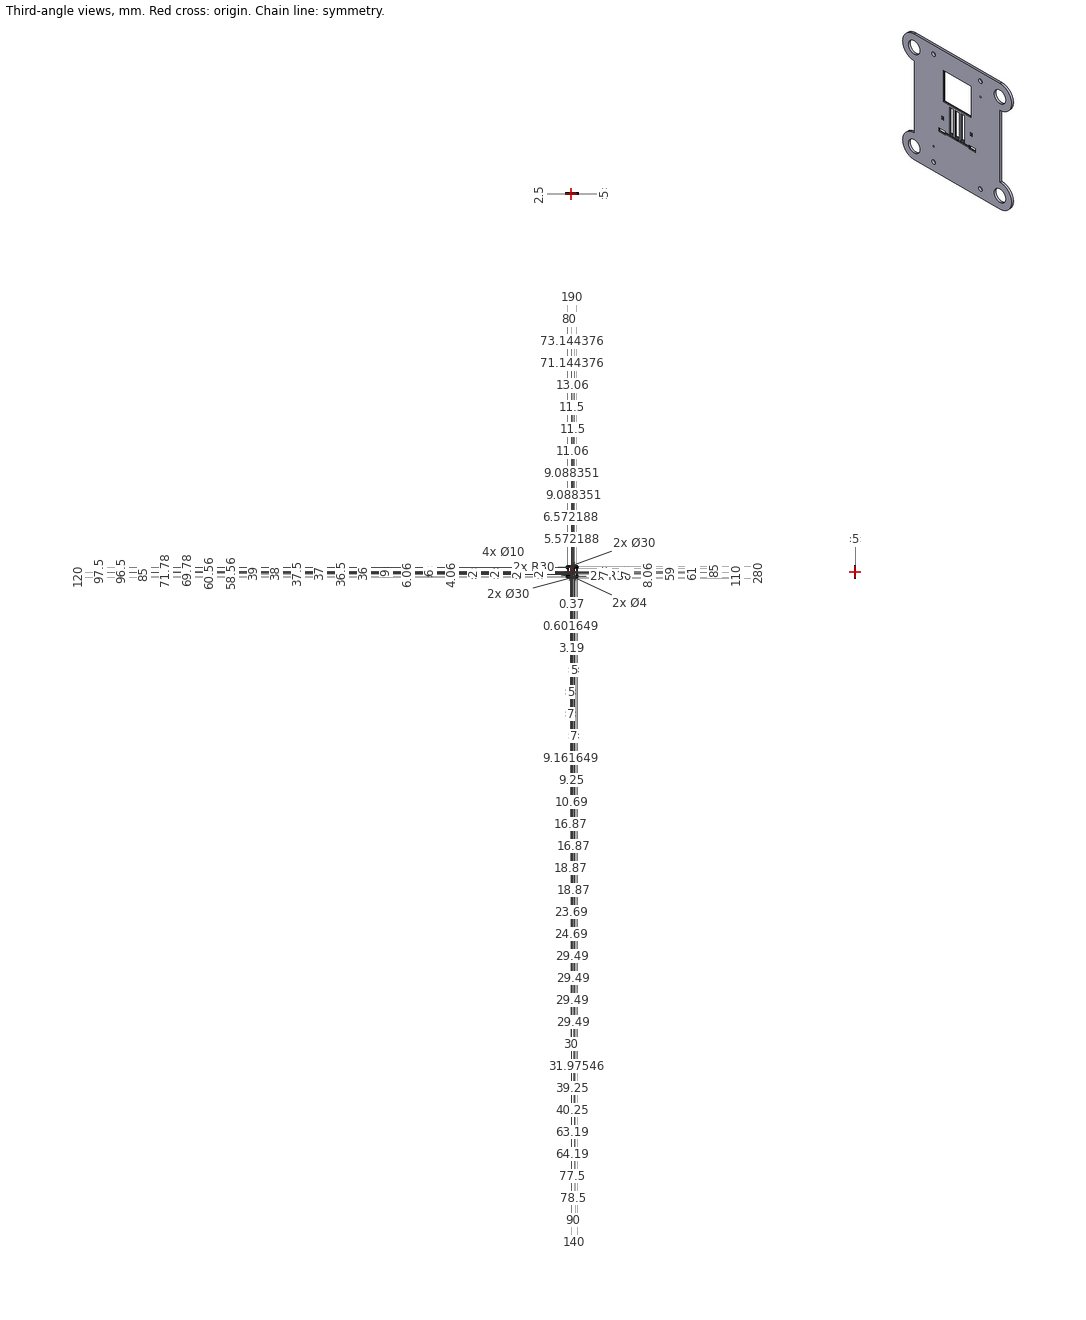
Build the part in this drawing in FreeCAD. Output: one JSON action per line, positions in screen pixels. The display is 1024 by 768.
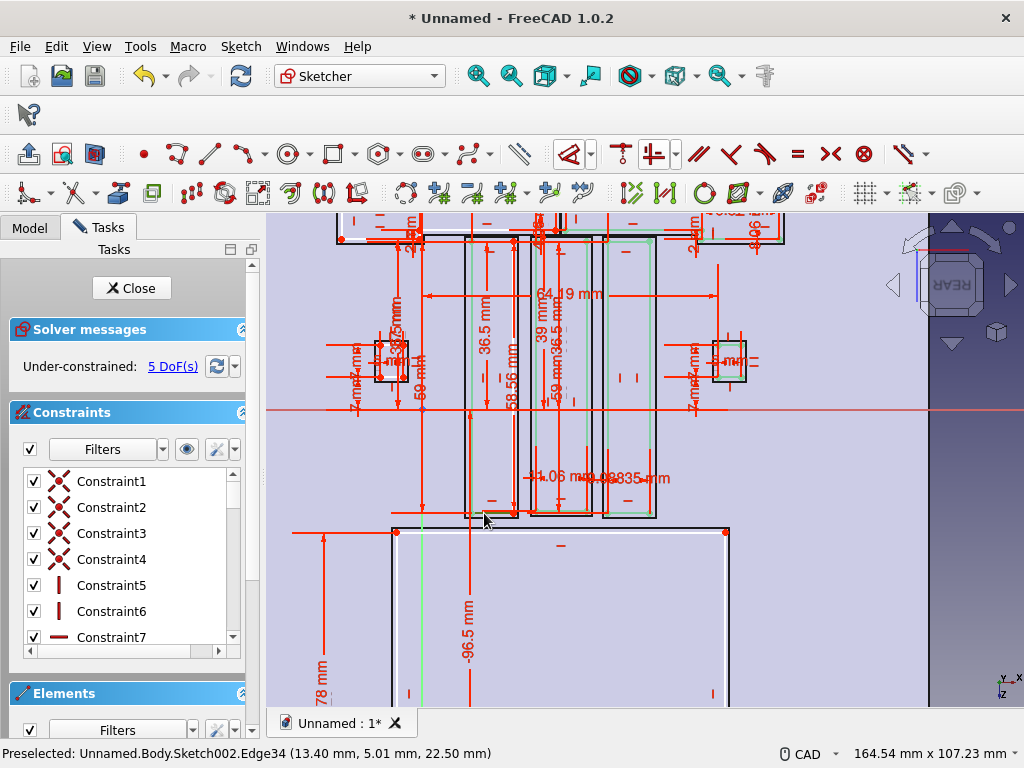
{"action": "key", "text": "l"}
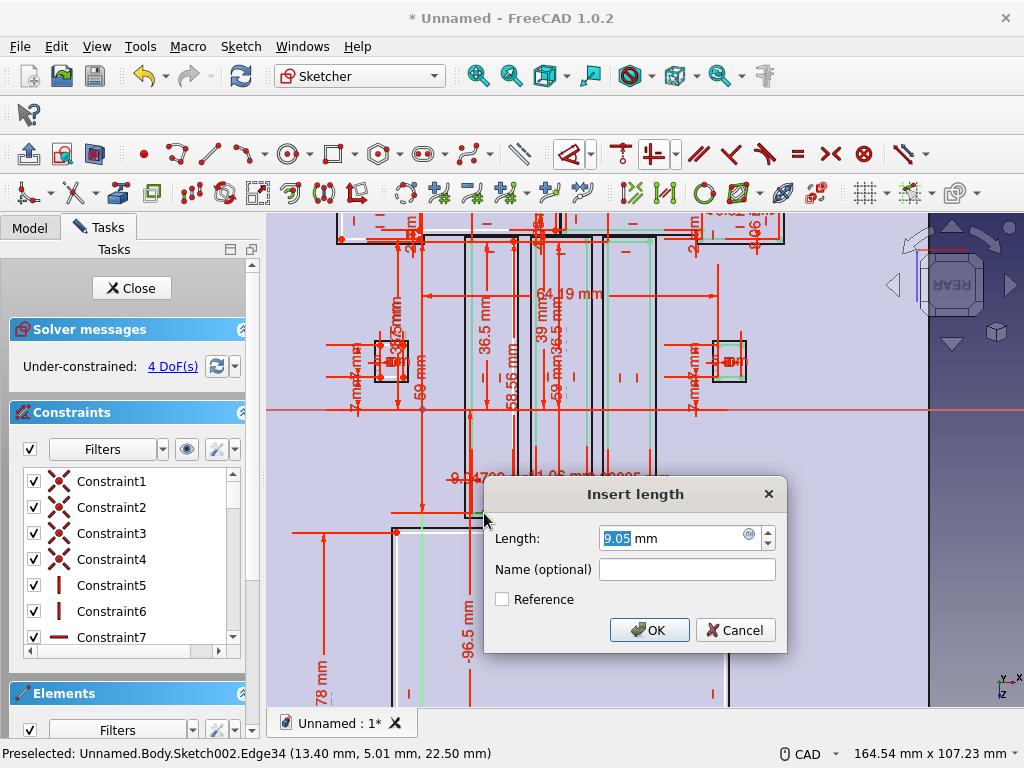
{"action": "type", "text": "9.088351"}
{"action": "key", "text": "Return"}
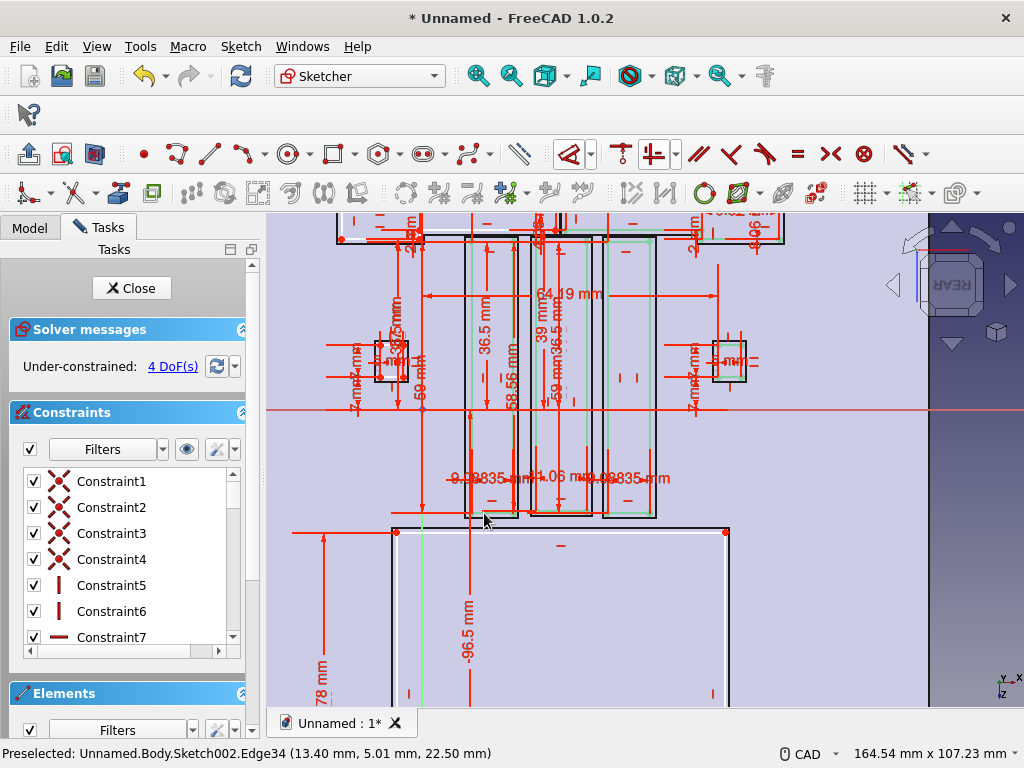
{"action": "scroll", "coordinate": [590, 404], "scroll_direction": "down", "scroll_amount": 4}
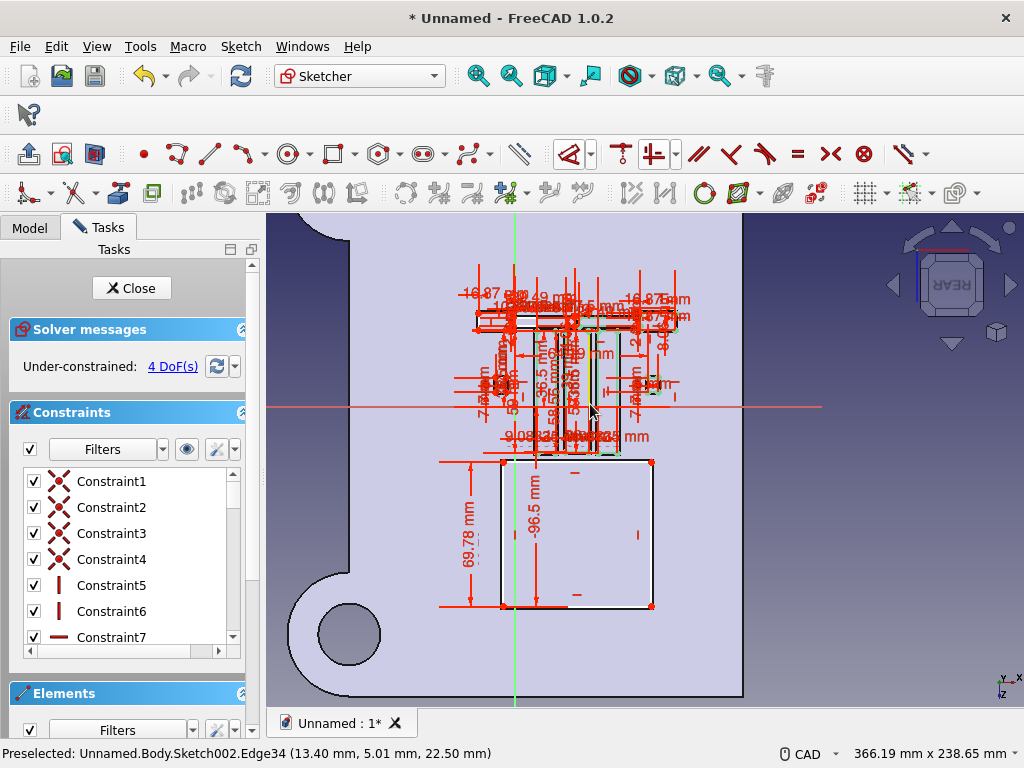
{"action": "left_click", "coordinate": [548, 607]}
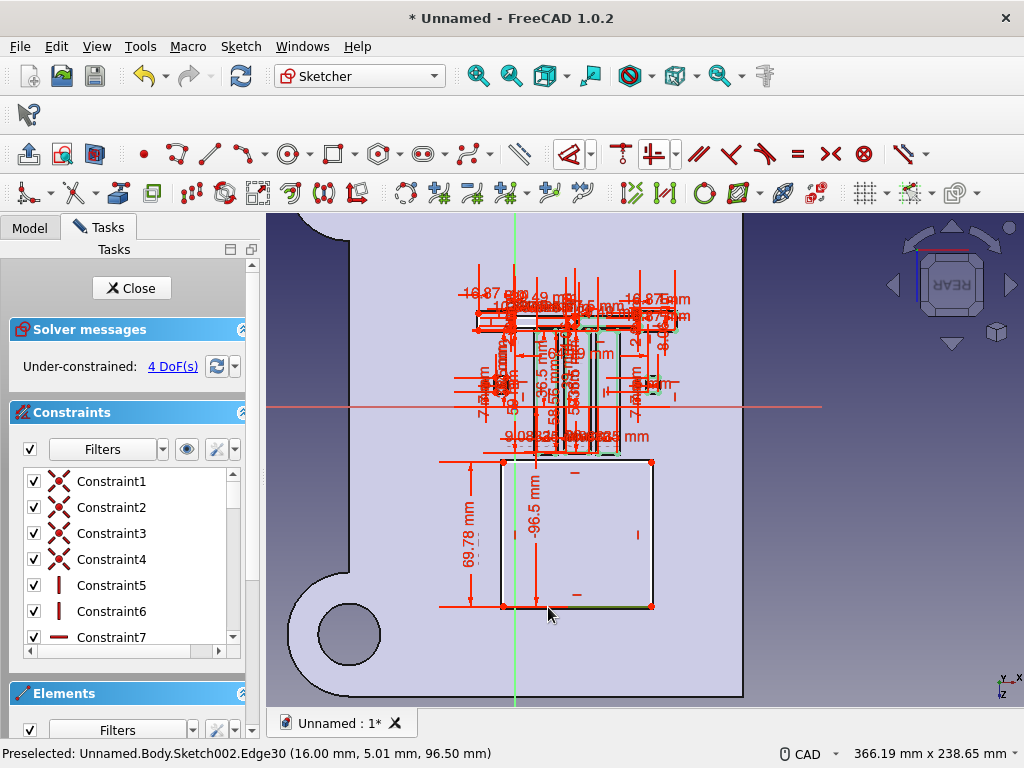
{"action": "key", "text": "l"}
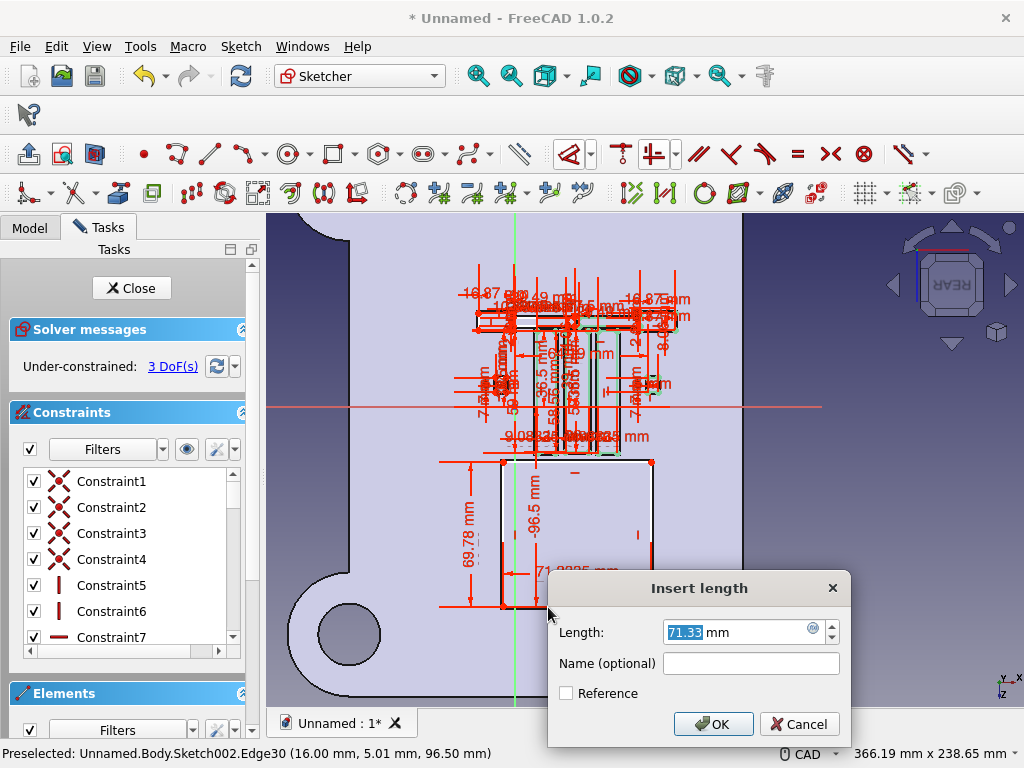
{"action": "type", "text": "71.144376"}
{"action": "key", "text": "Return"}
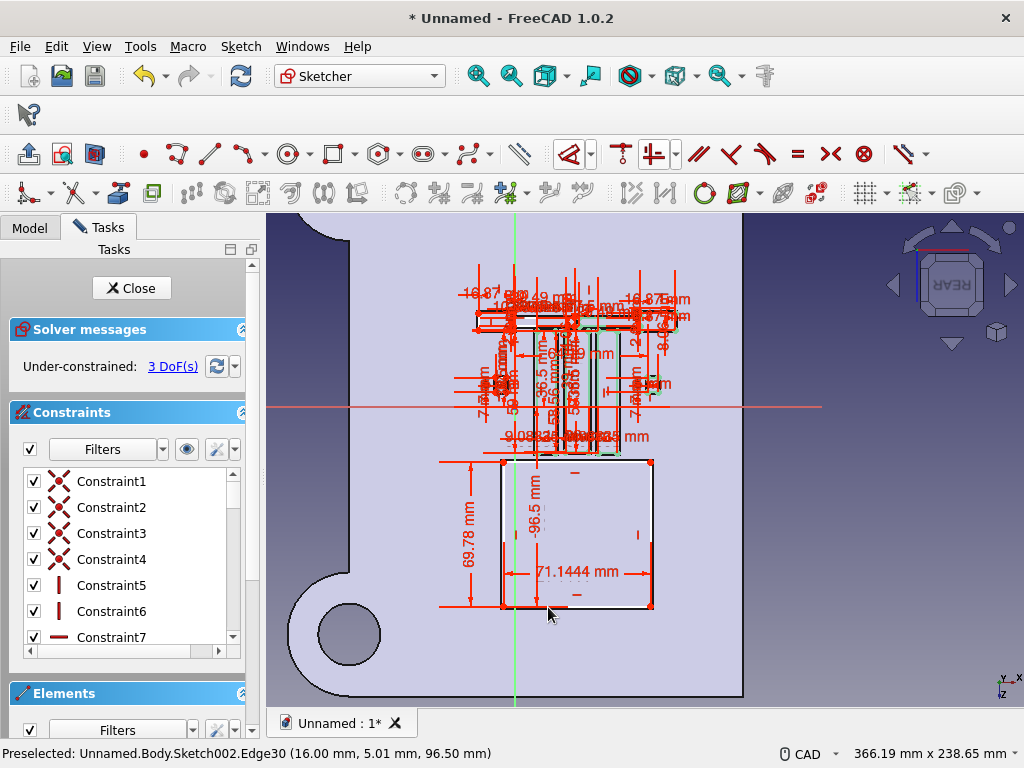
{"action": "scroll", "coordinate": [514, 330], "scroll_direction": "up", "scroll_amount": 18}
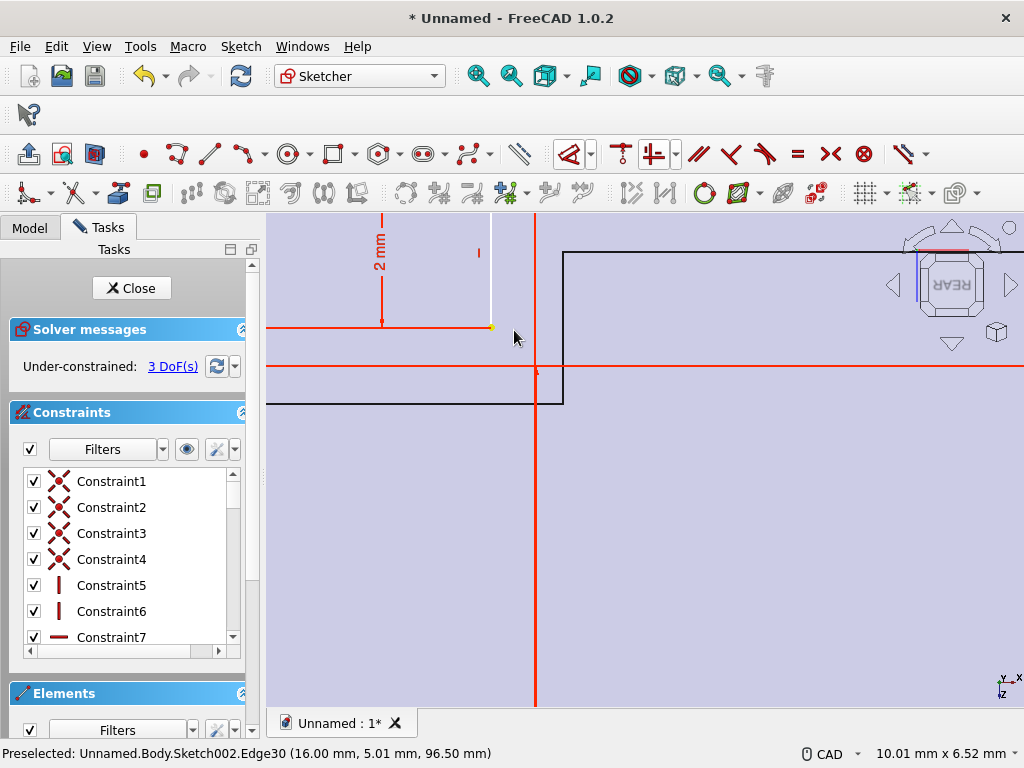
{"action": "left_click", "coordinate": [491, 328]}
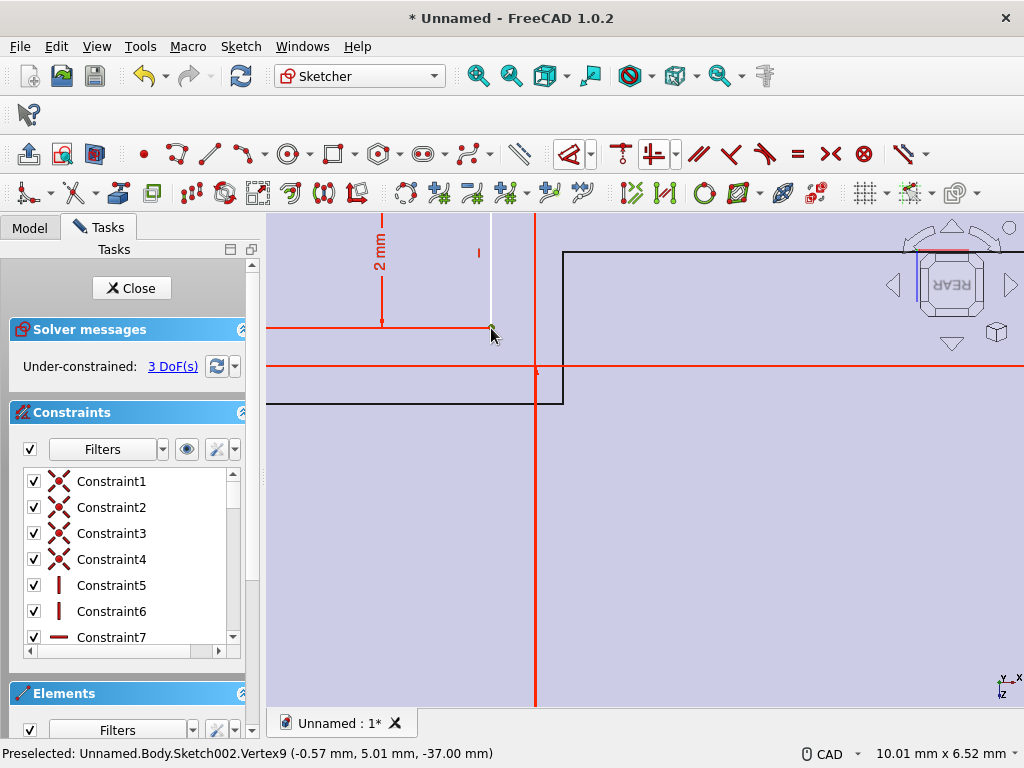
{"action": "left_click", "coordinate": [590, 154]}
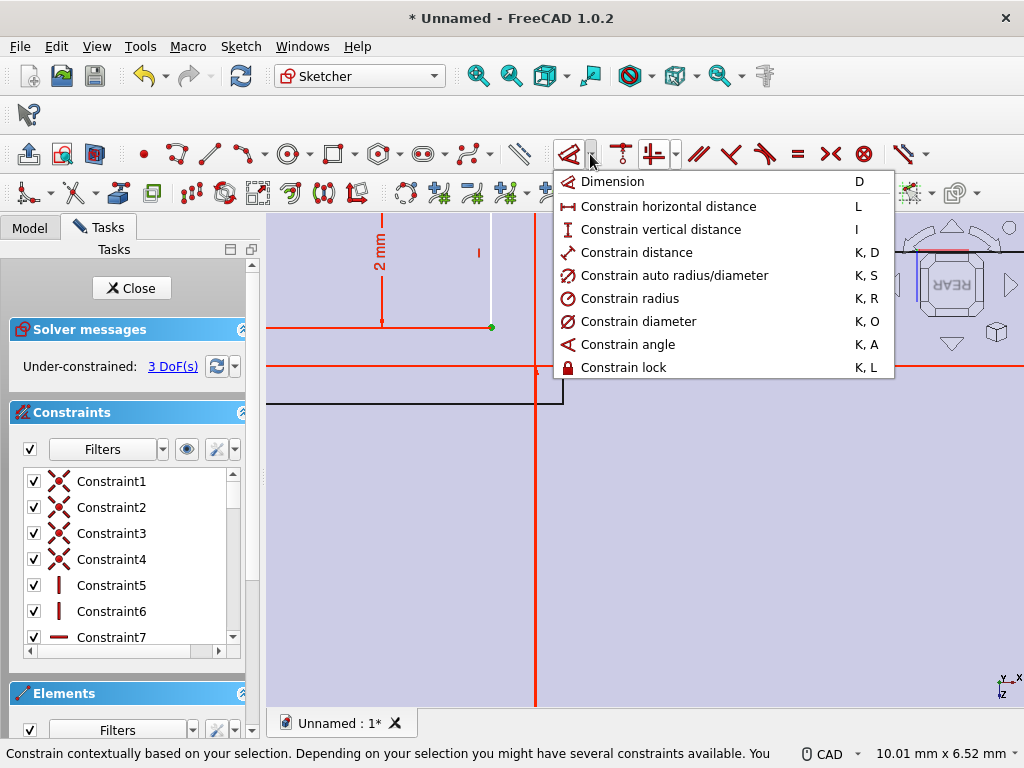
{"action": "left_click", "coordinate": [724, 206]}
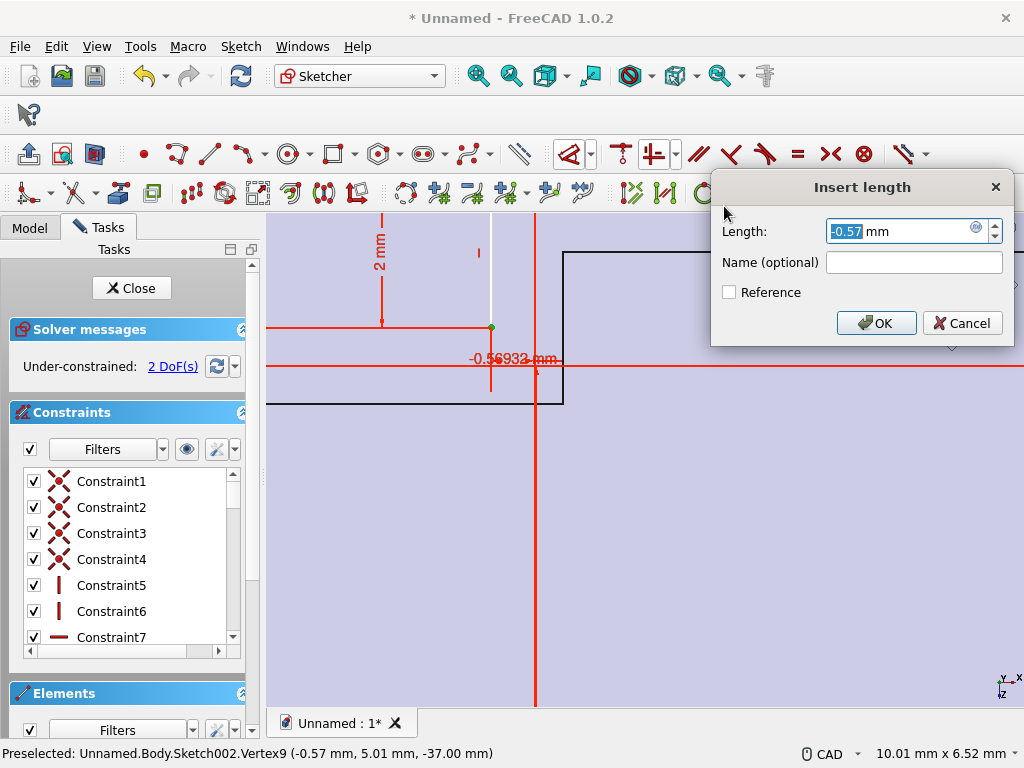
{"action": "type", "text": "-0.601649"}
{"action": "key", "text": "Return"}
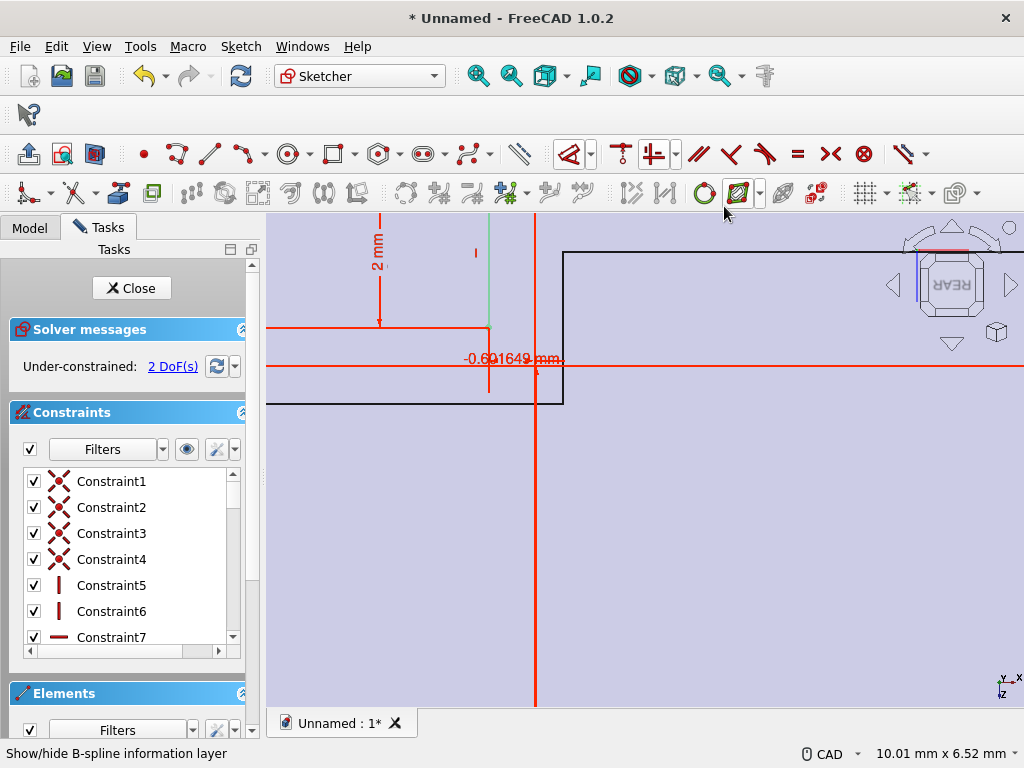
{"action": "scroll", "coordinate": [499, 301], "scroll_direction": "down", "scroll_amount": 17}